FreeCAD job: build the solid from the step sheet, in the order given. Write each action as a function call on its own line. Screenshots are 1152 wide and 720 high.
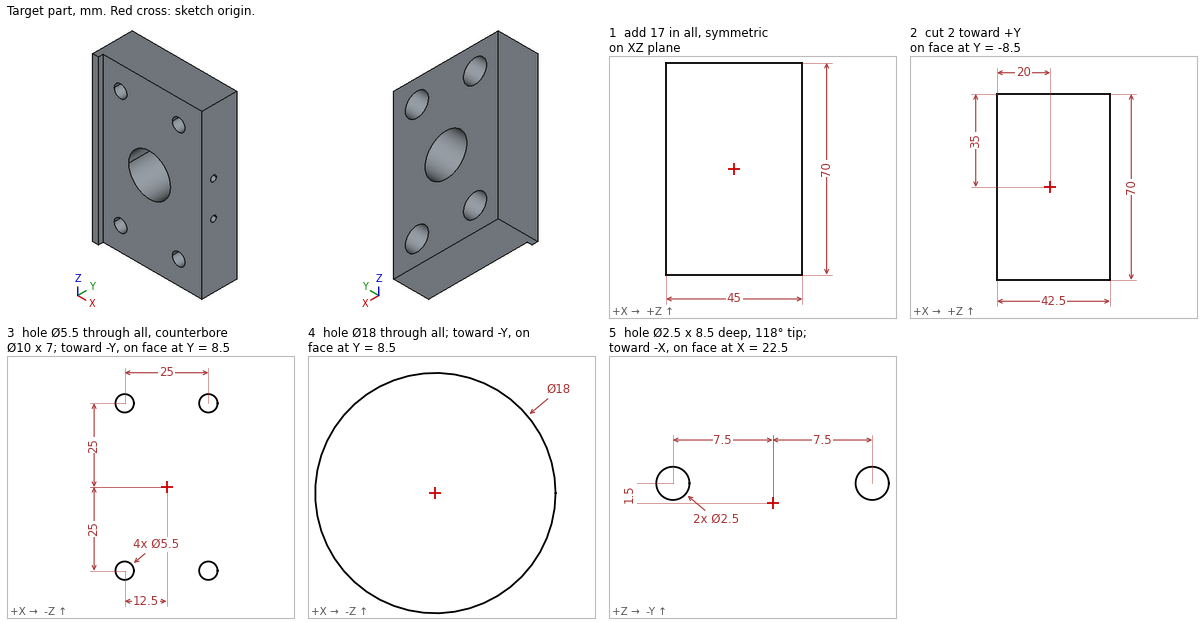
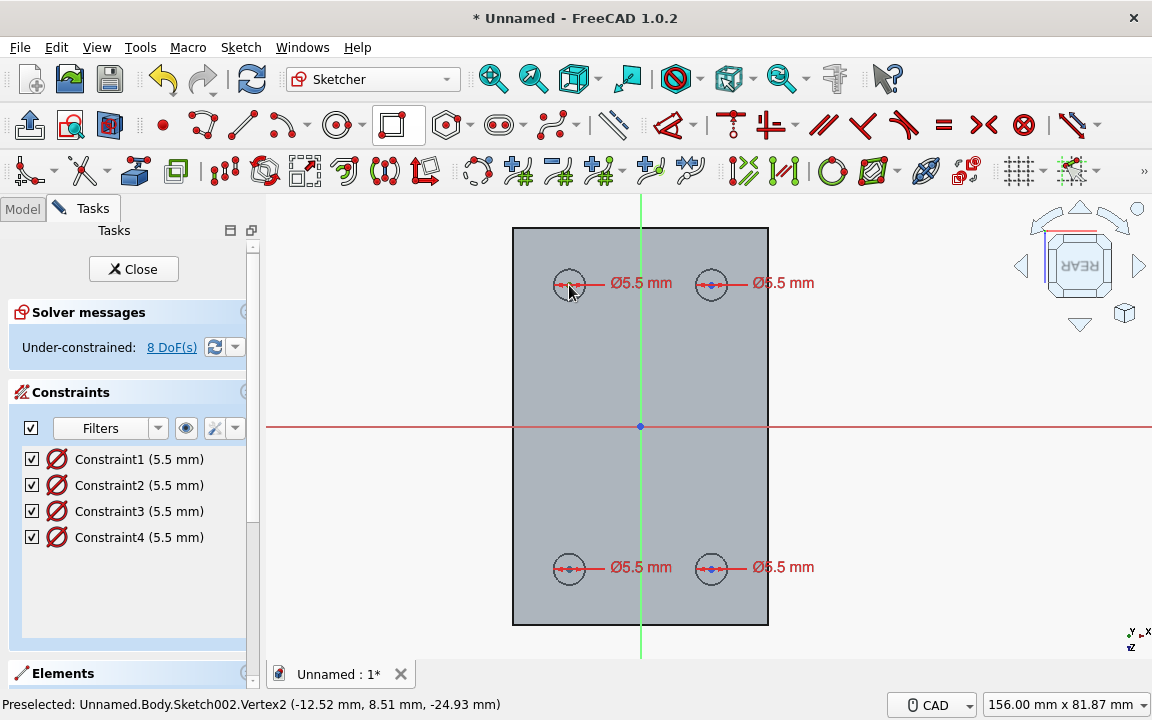
click(798, 126)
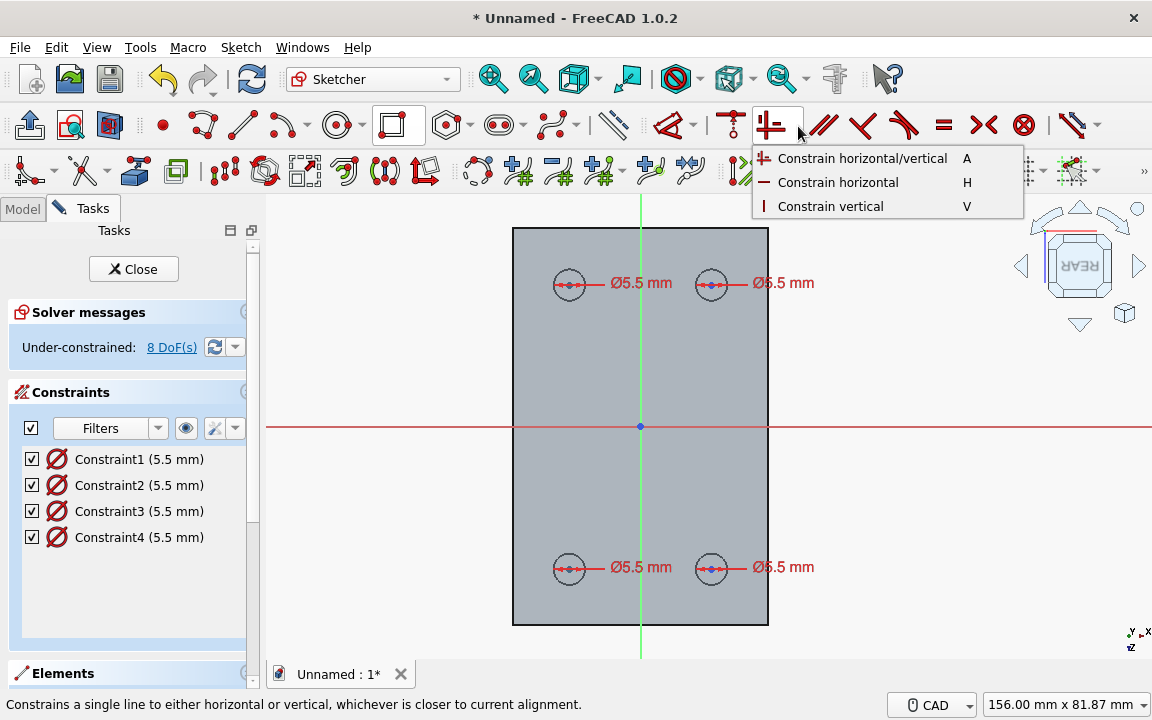
click(888, 206)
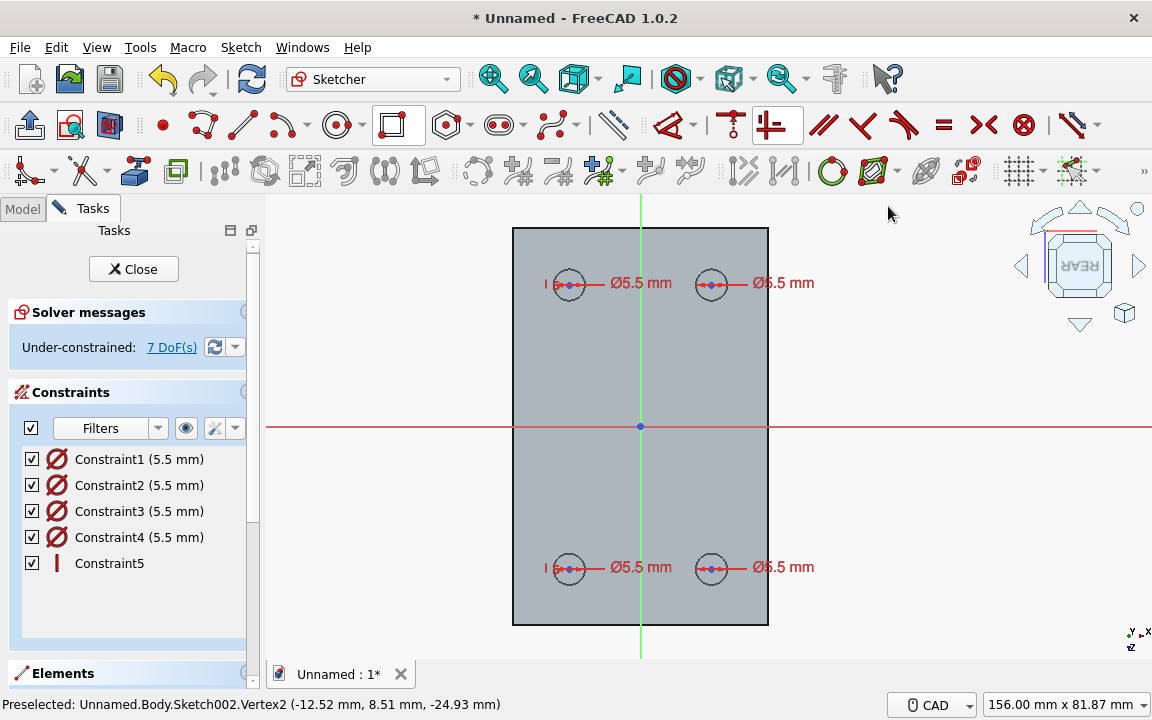
click(569, 285)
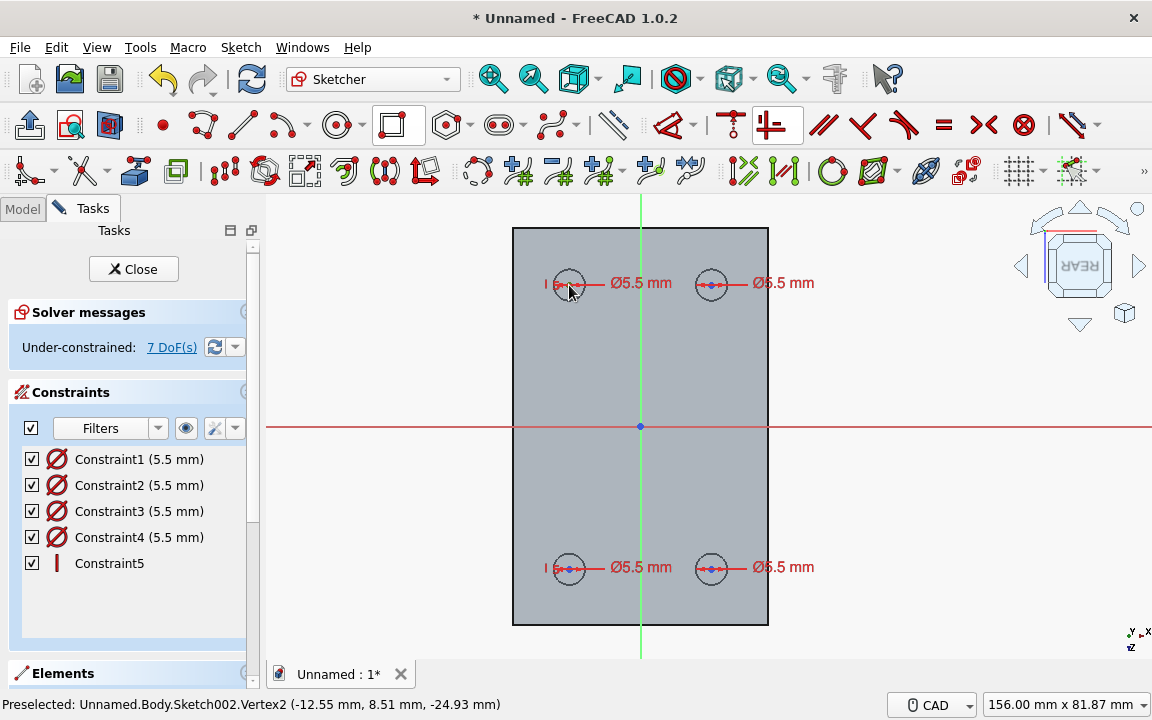
click(712, 285)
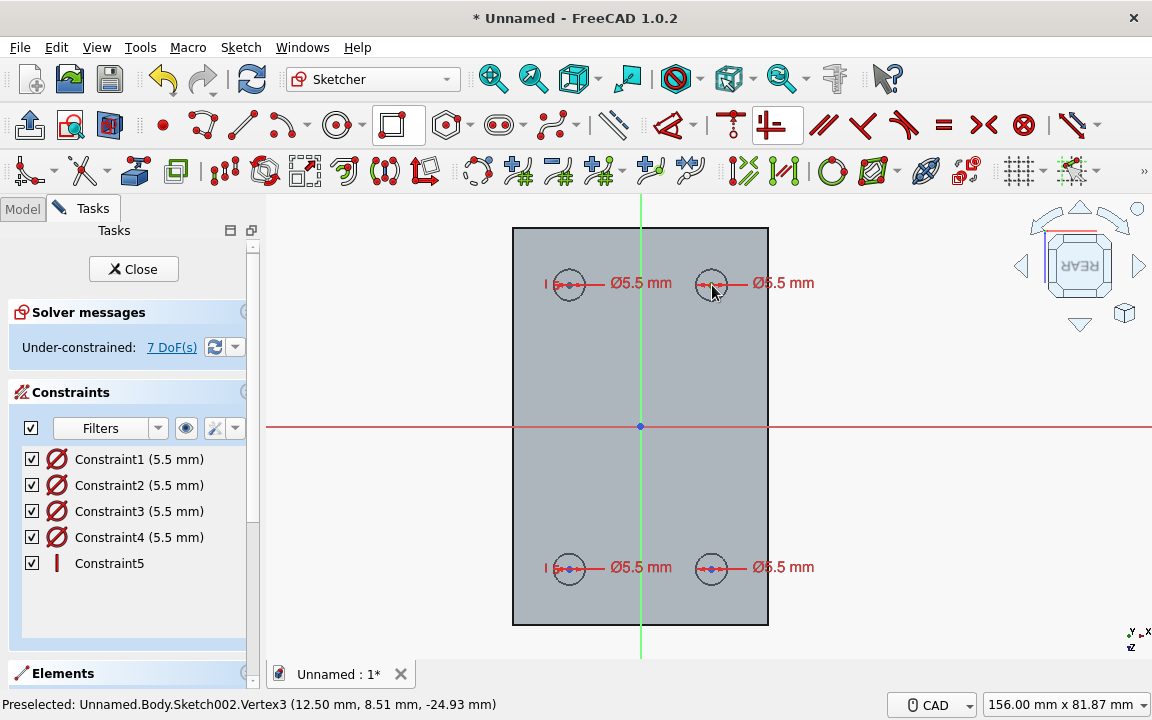
click(798, 126)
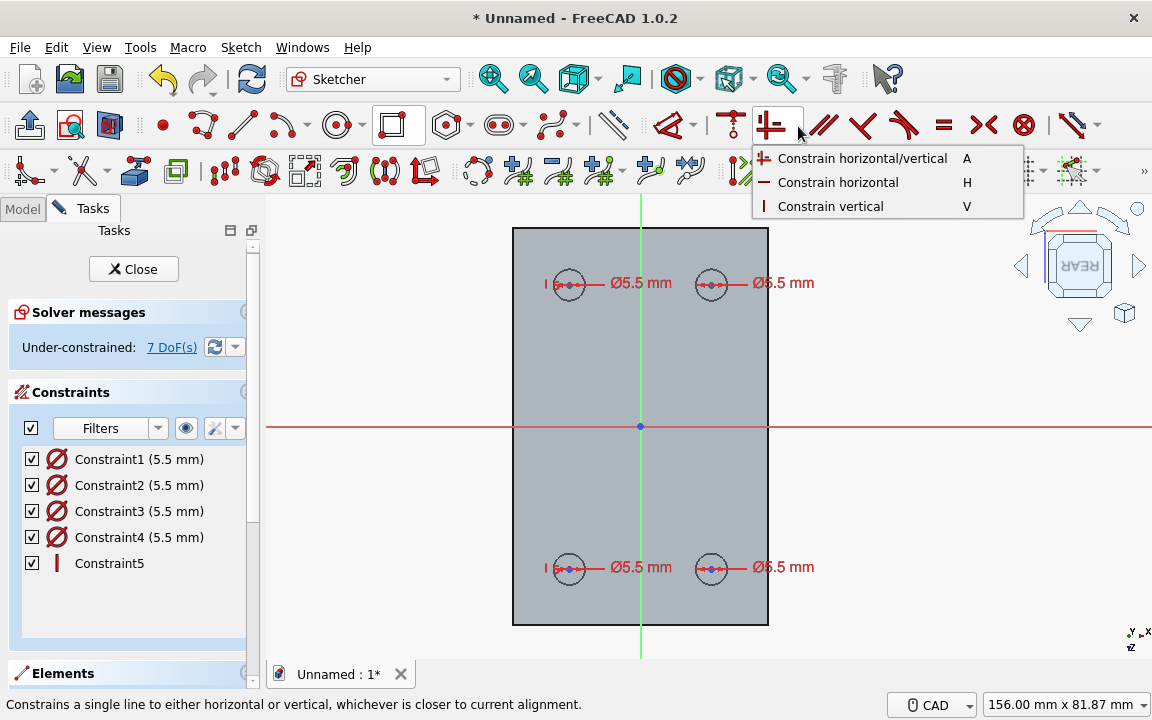
click(888, 182)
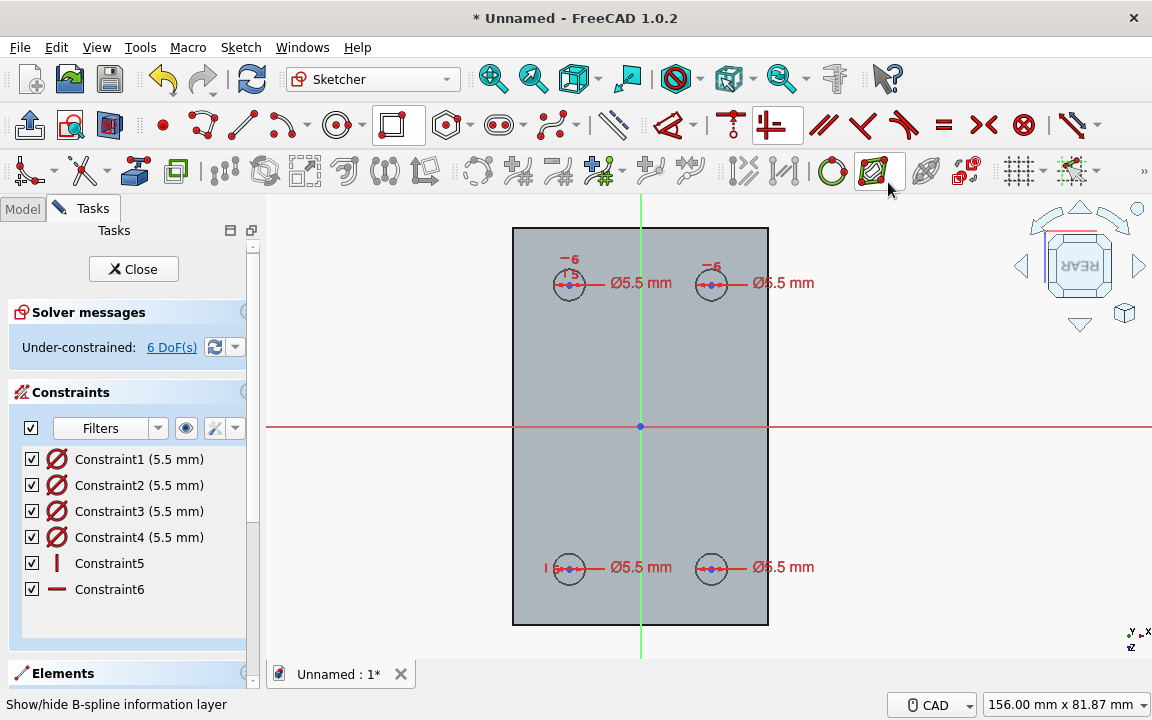
click(712, 285)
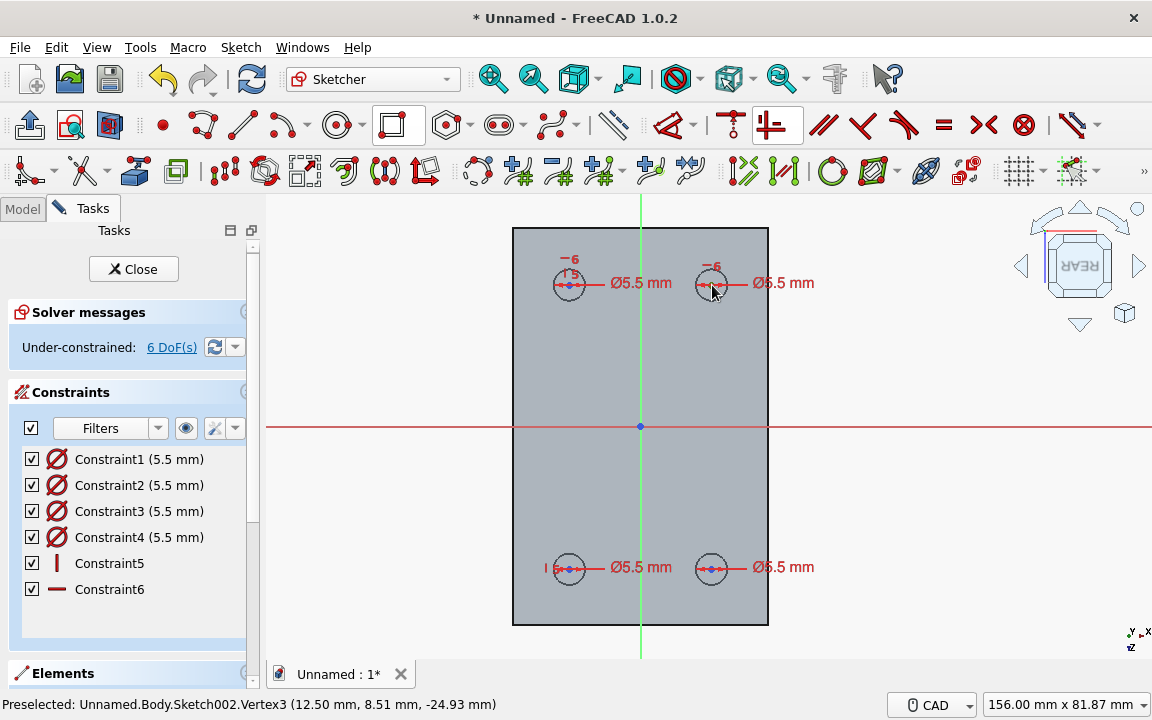
click(711, 569)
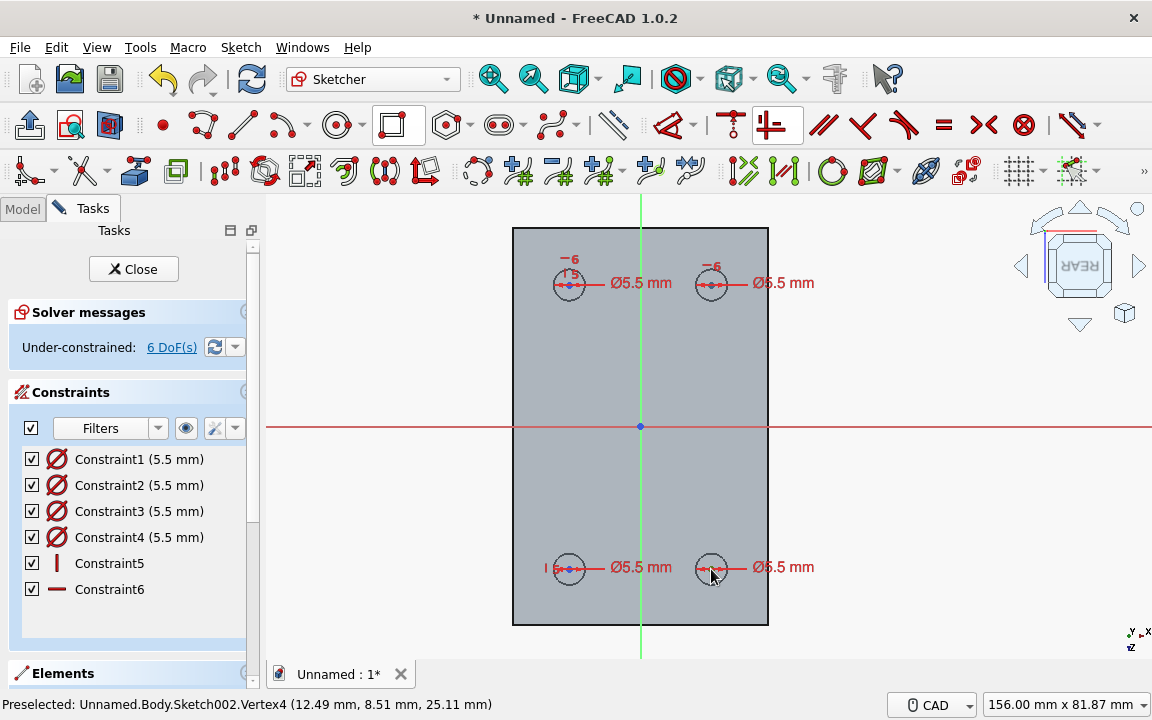
click(798, 126)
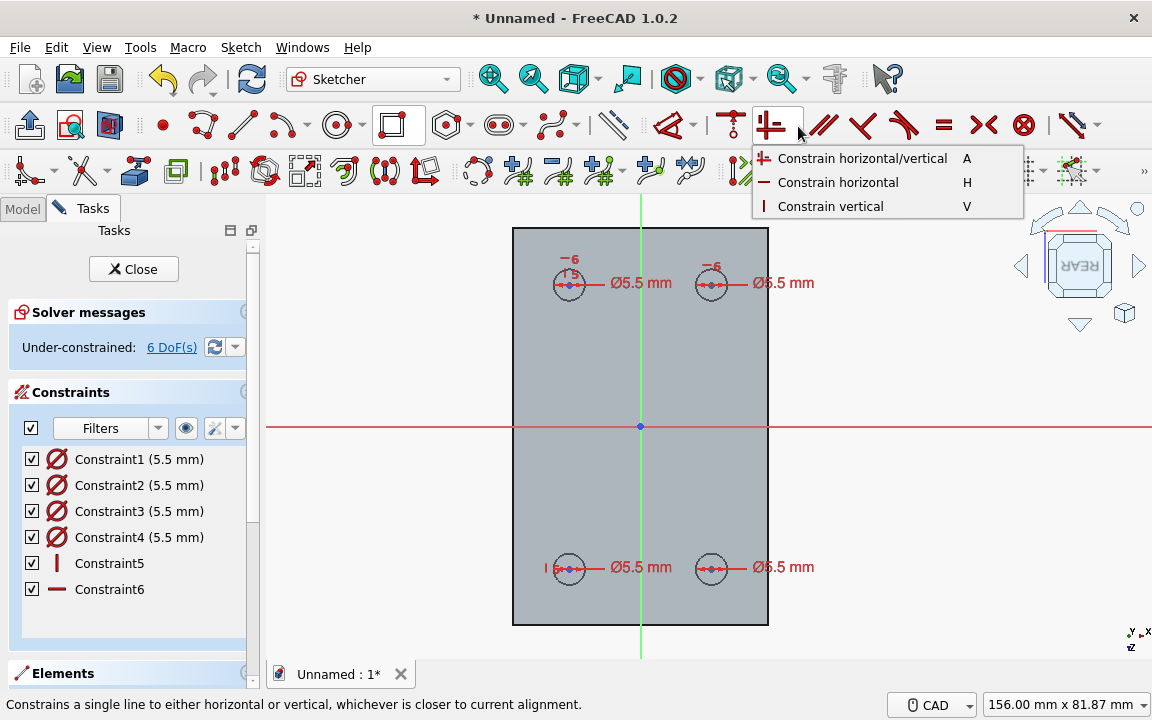
click(888, 206)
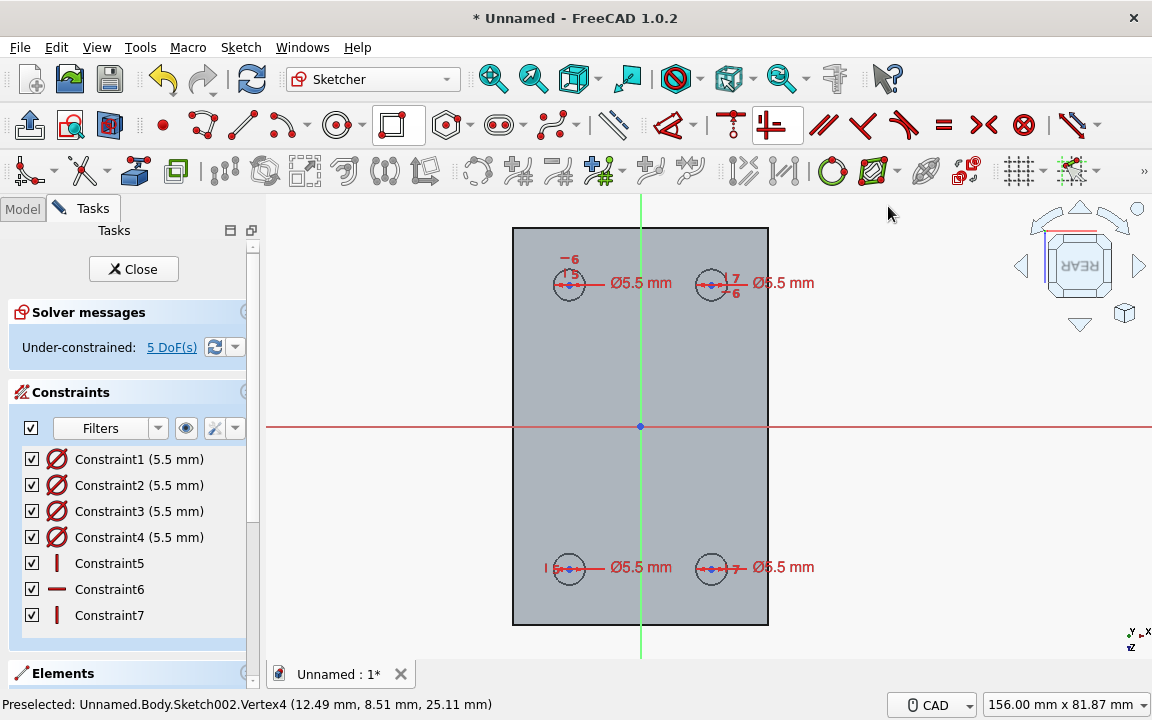
click(569, 569)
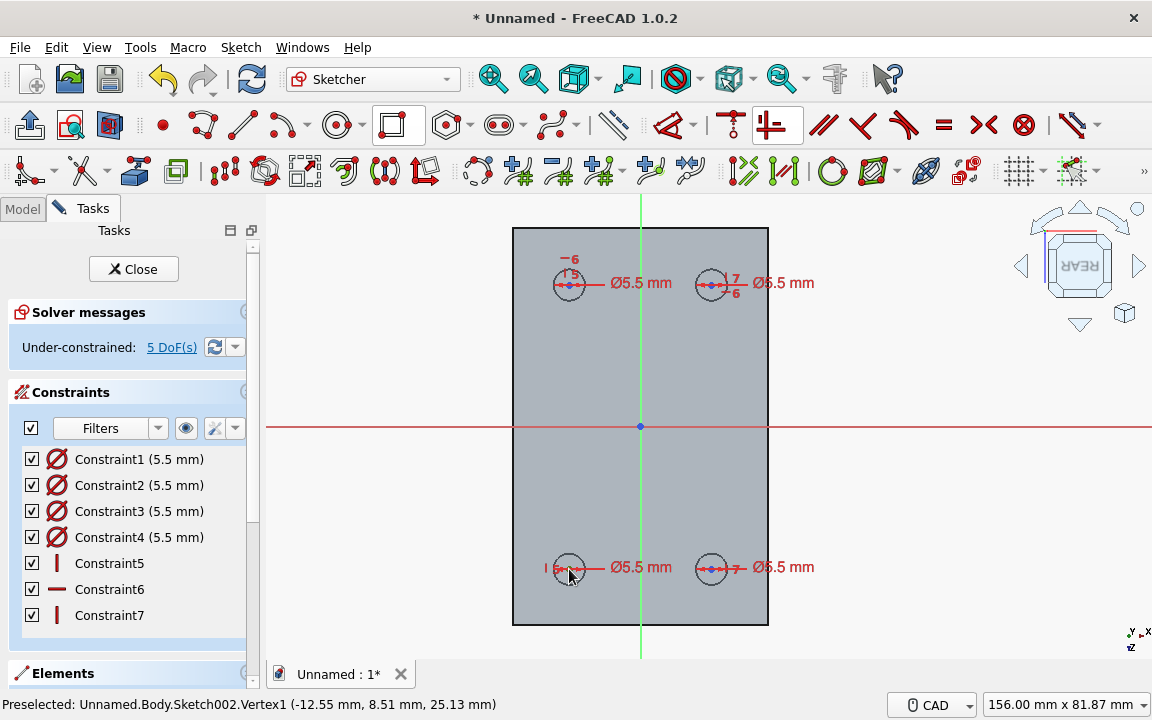
click(712, 569)